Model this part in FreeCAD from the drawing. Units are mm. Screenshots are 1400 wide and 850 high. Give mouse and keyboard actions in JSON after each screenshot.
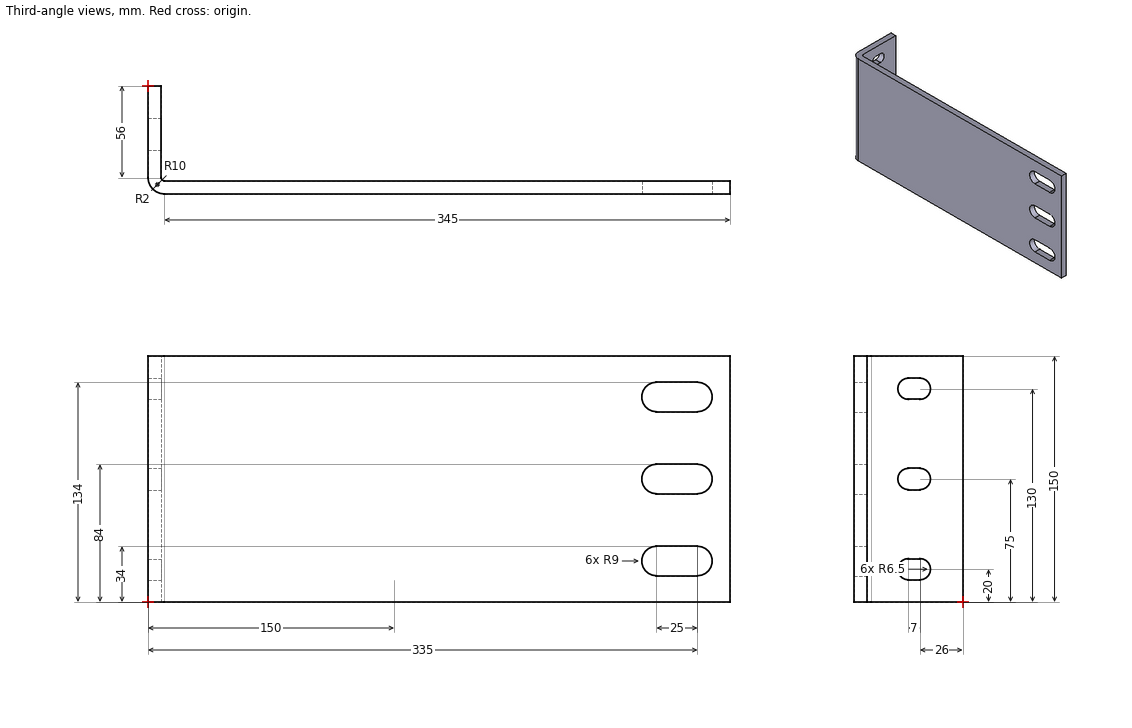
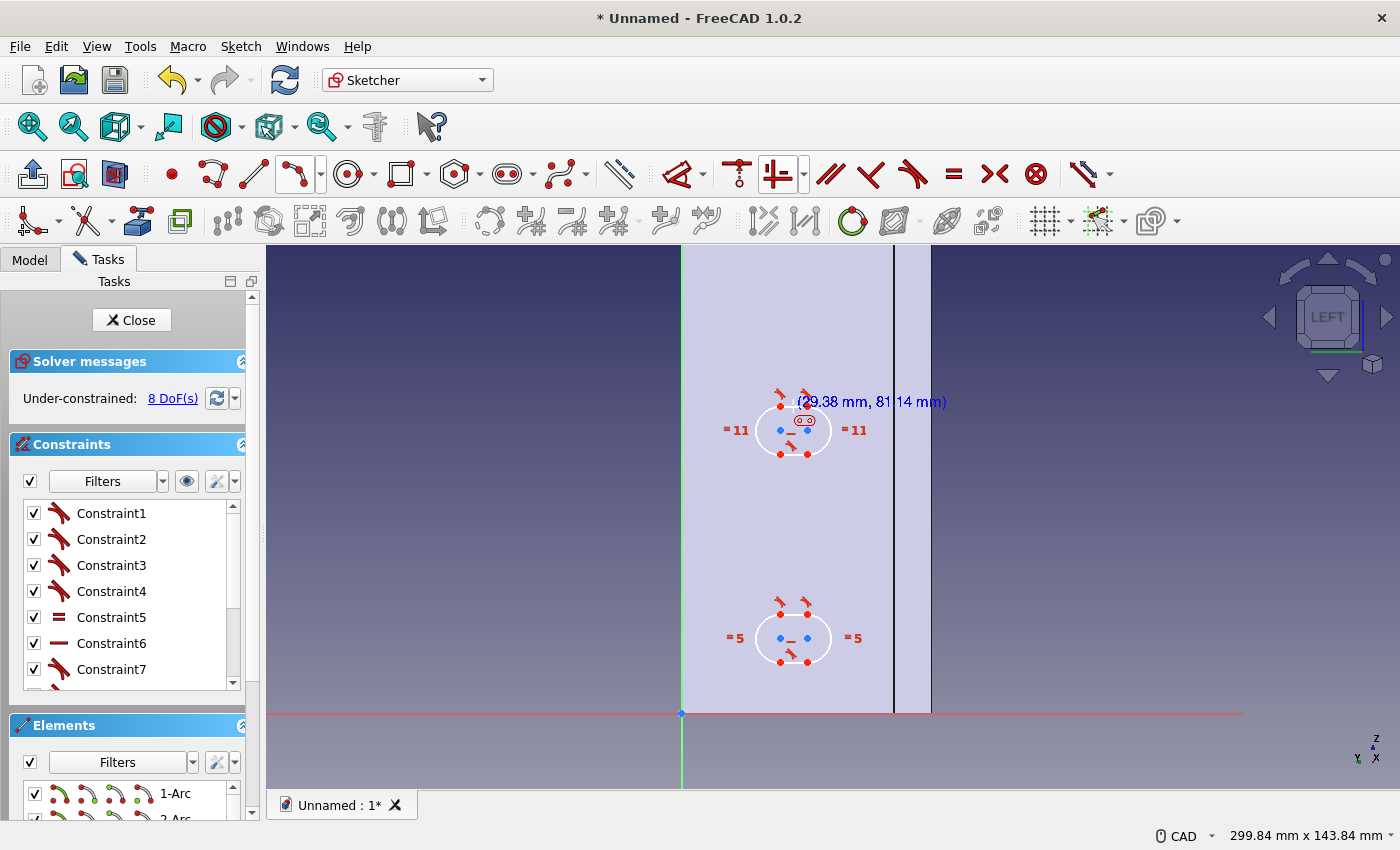
{"action": "scroll", "coordinate": [781, 642], "scroll_direction": "down", "scroll_amount": 2}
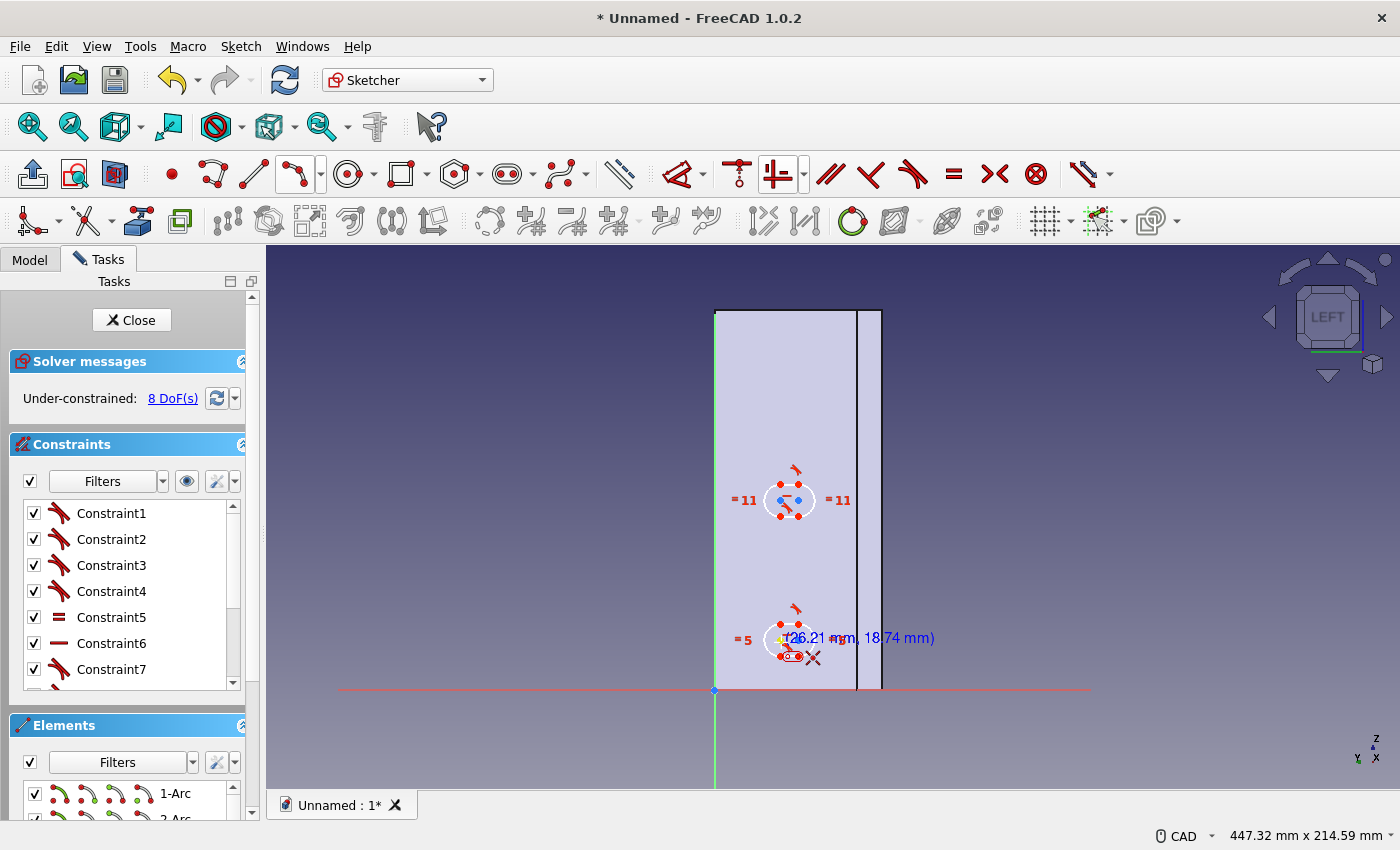
{"action": "scroll", "coordinate": [781, 361], "scroll_direction": "up", "scroll_amount": 2}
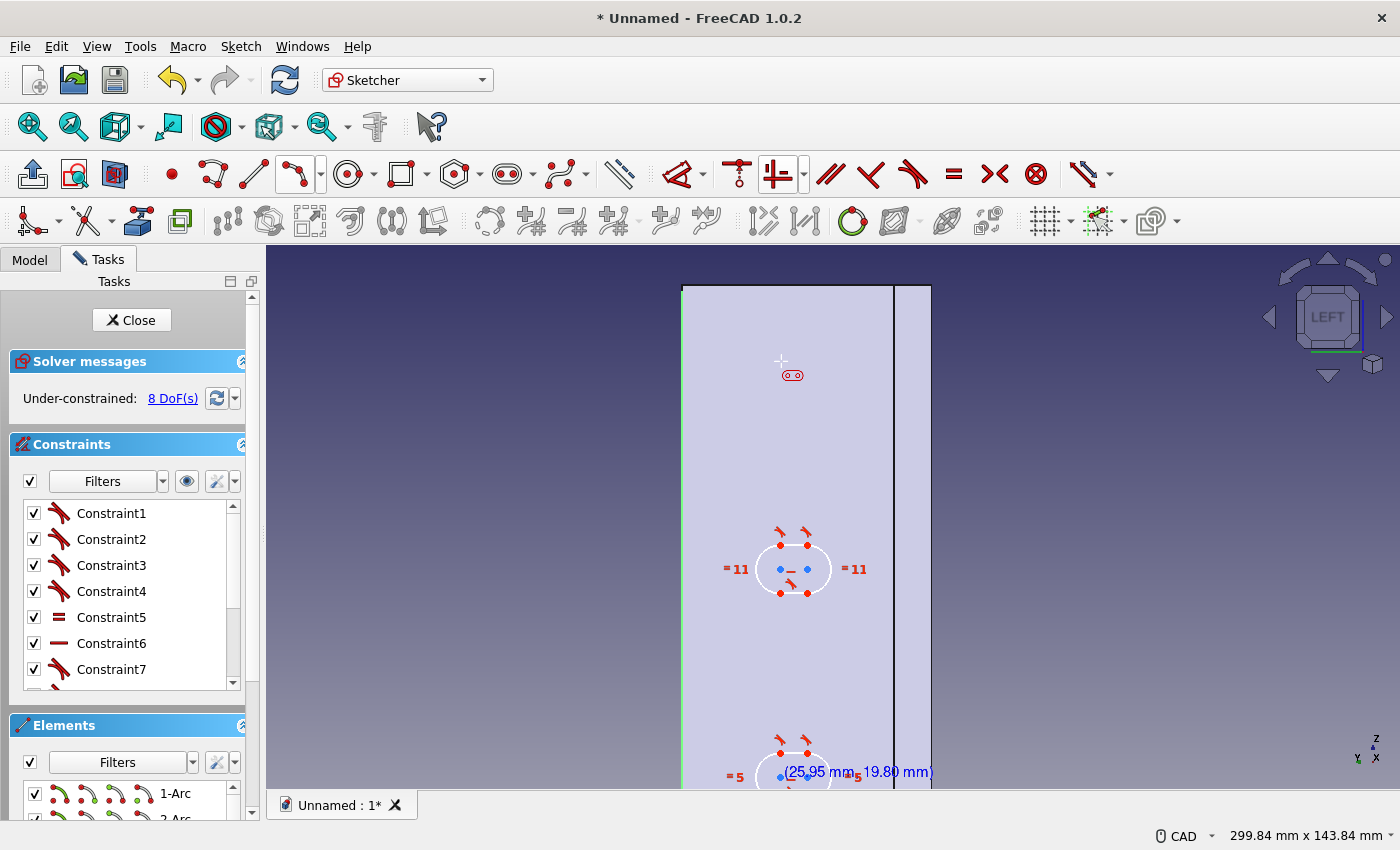
{"action": "left_click", "coordinate": [780, 361]}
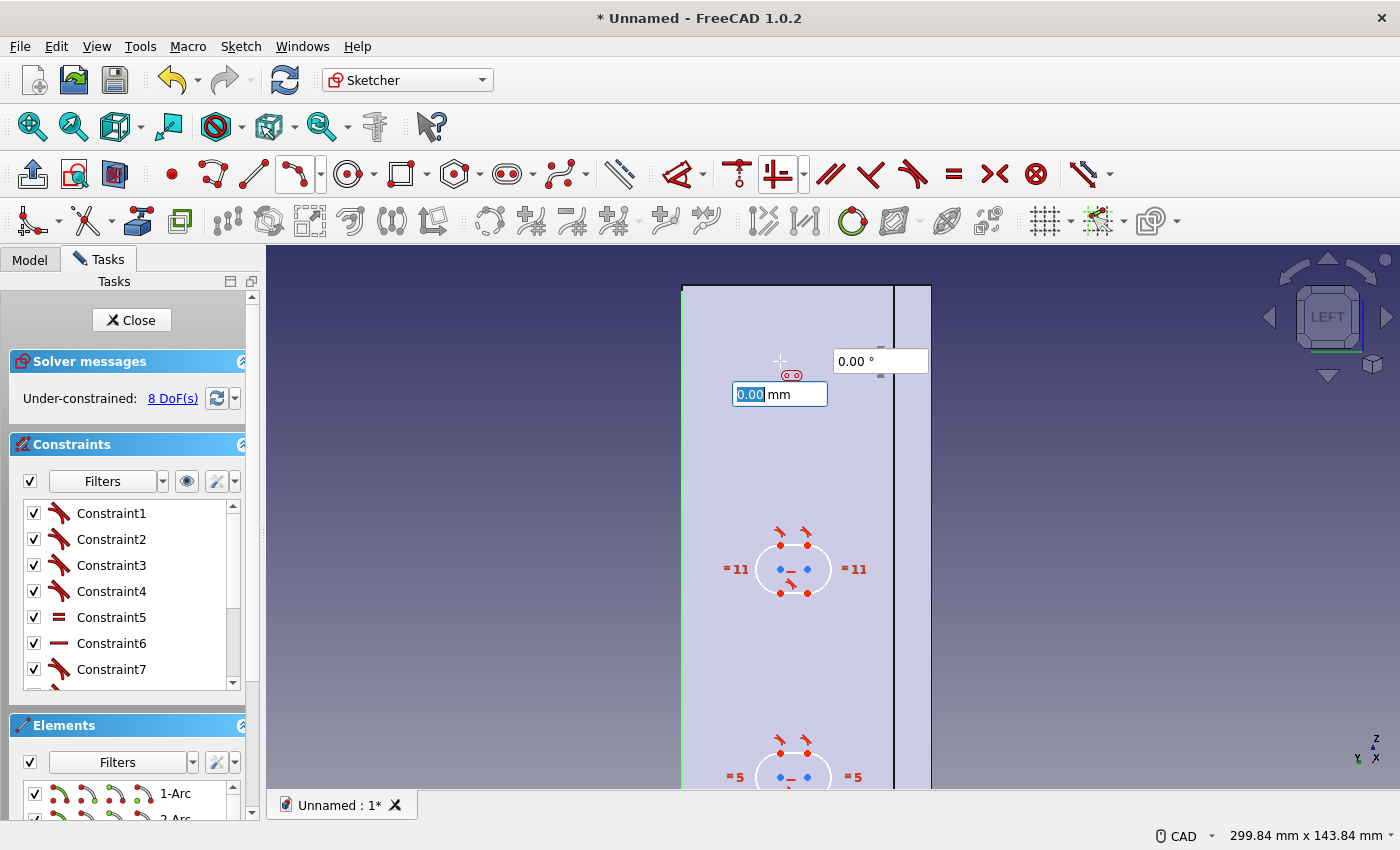
{"action": "left_click", "coordinate": [807, 361]}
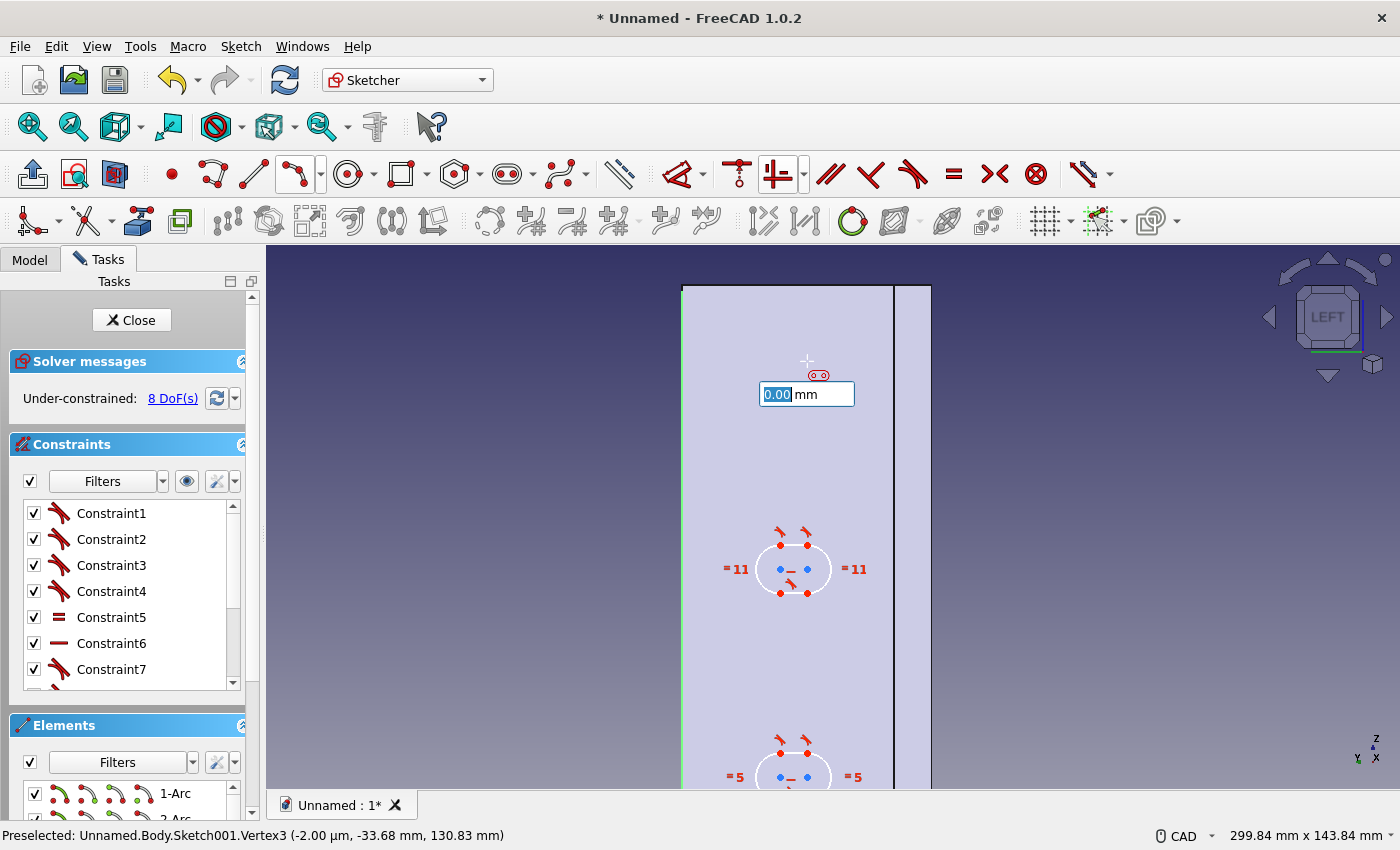
{"action": "left_click", "coordinate": [793, 336]}
{"action": "key", "text": "Escape"}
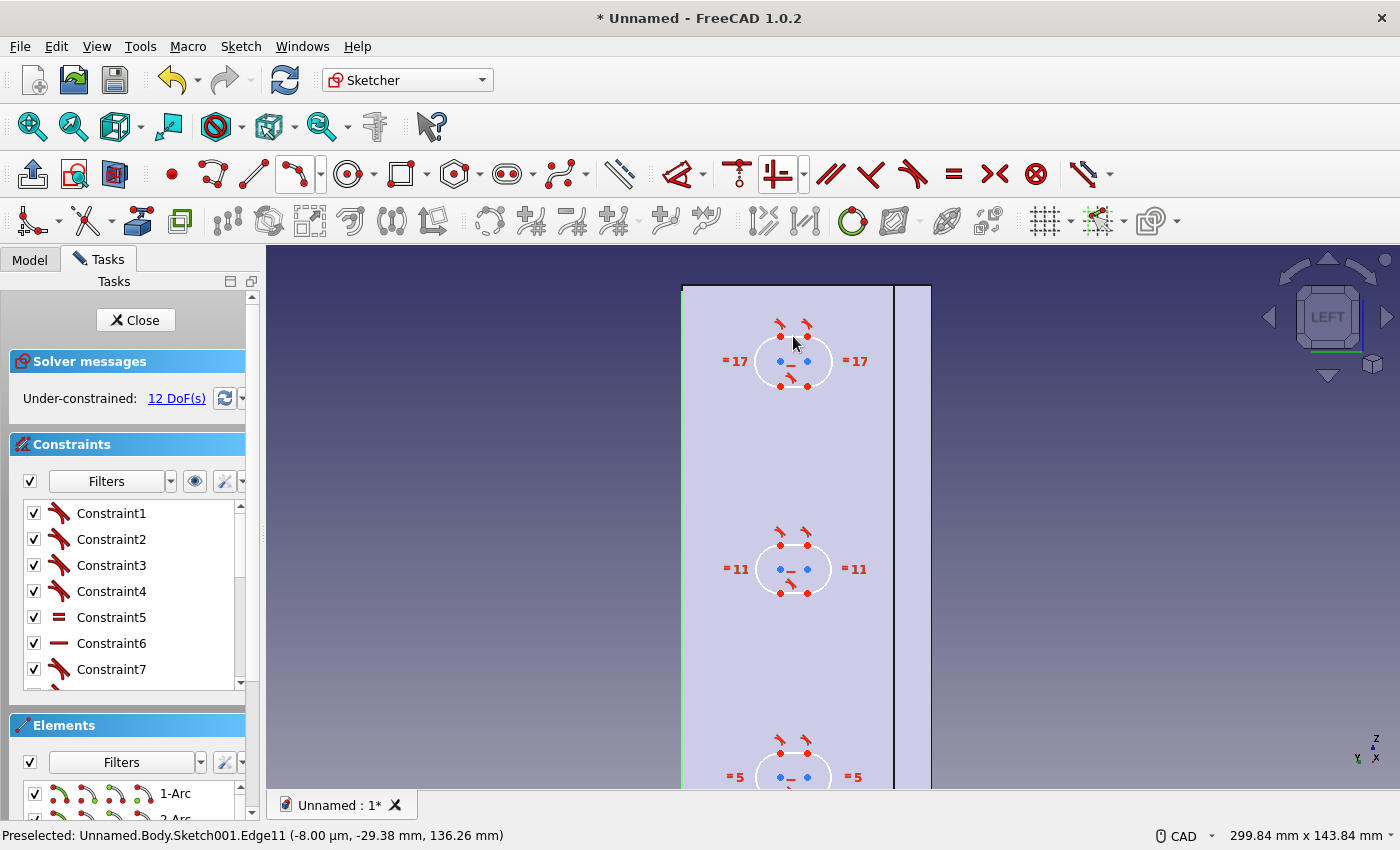
{"action": "left_click", "coordinate": [766, 758]}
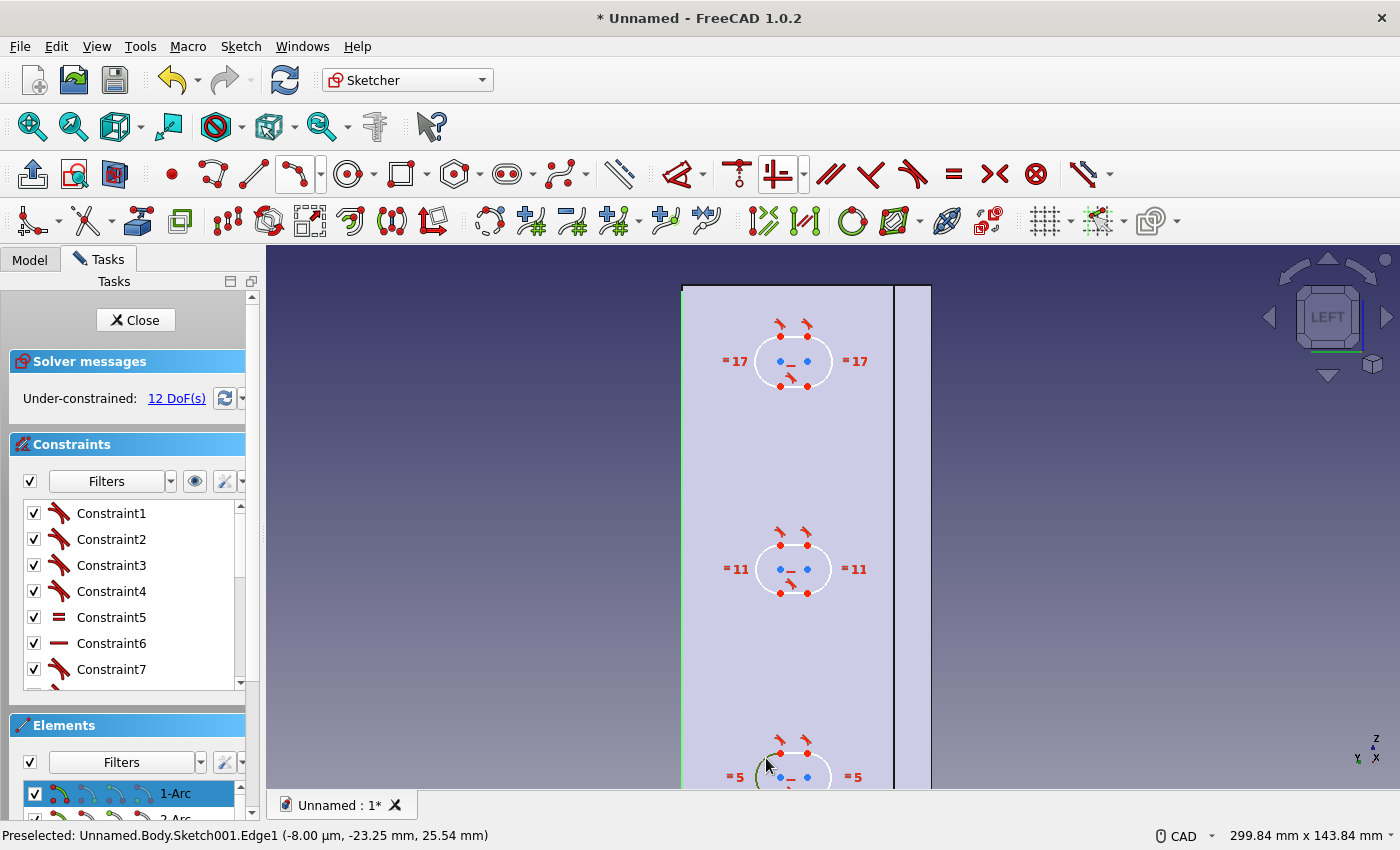
{"action": "left_click", "coordinate": [761, 555]}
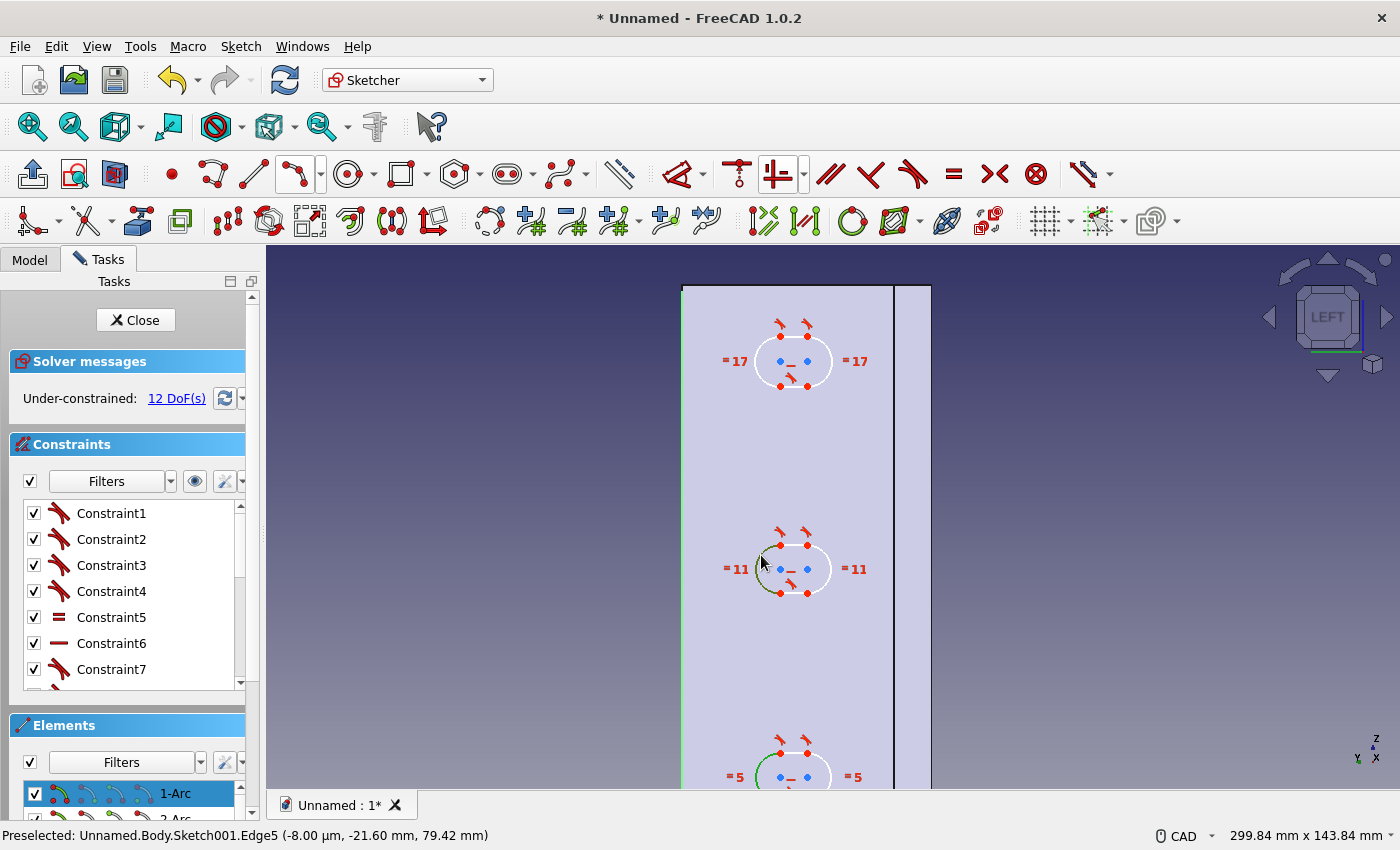
{"action": "left_click", "coordinate": [760, 347]}